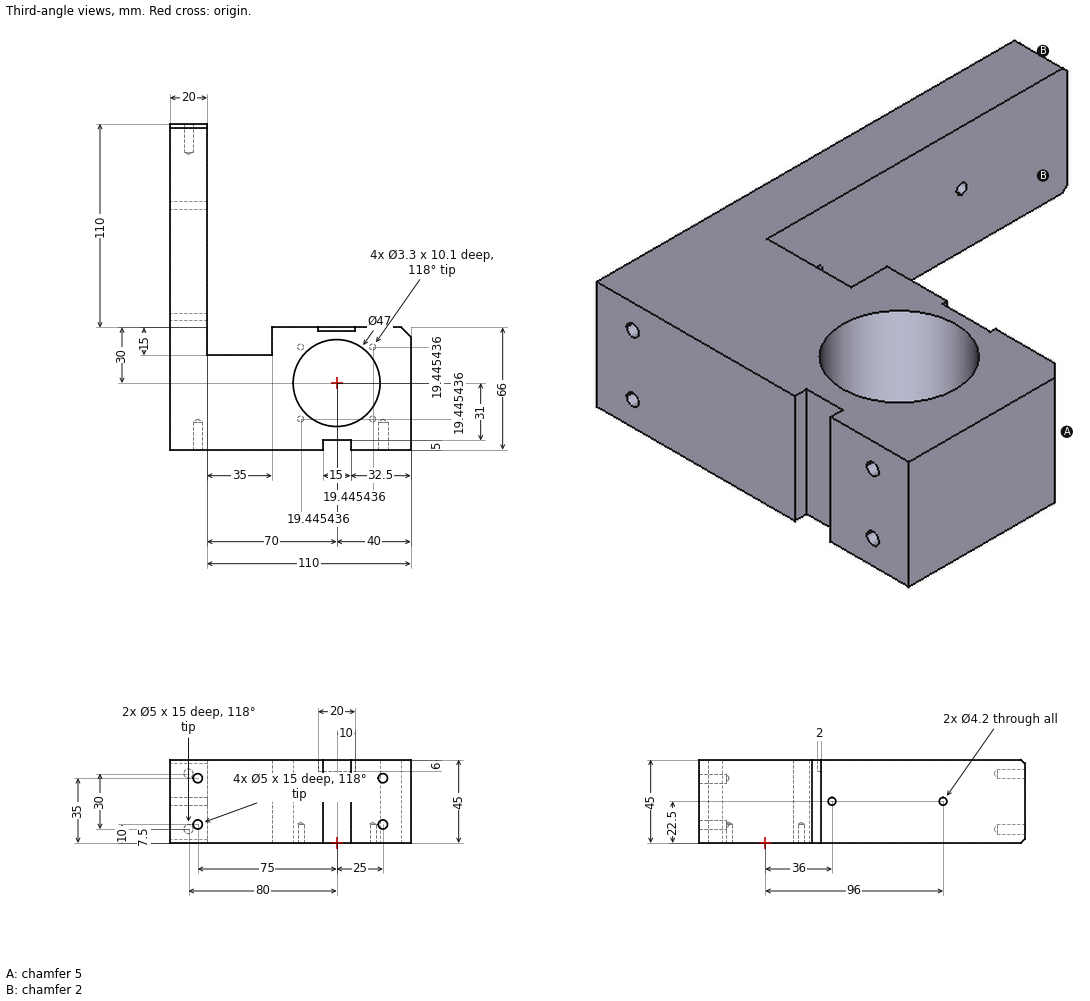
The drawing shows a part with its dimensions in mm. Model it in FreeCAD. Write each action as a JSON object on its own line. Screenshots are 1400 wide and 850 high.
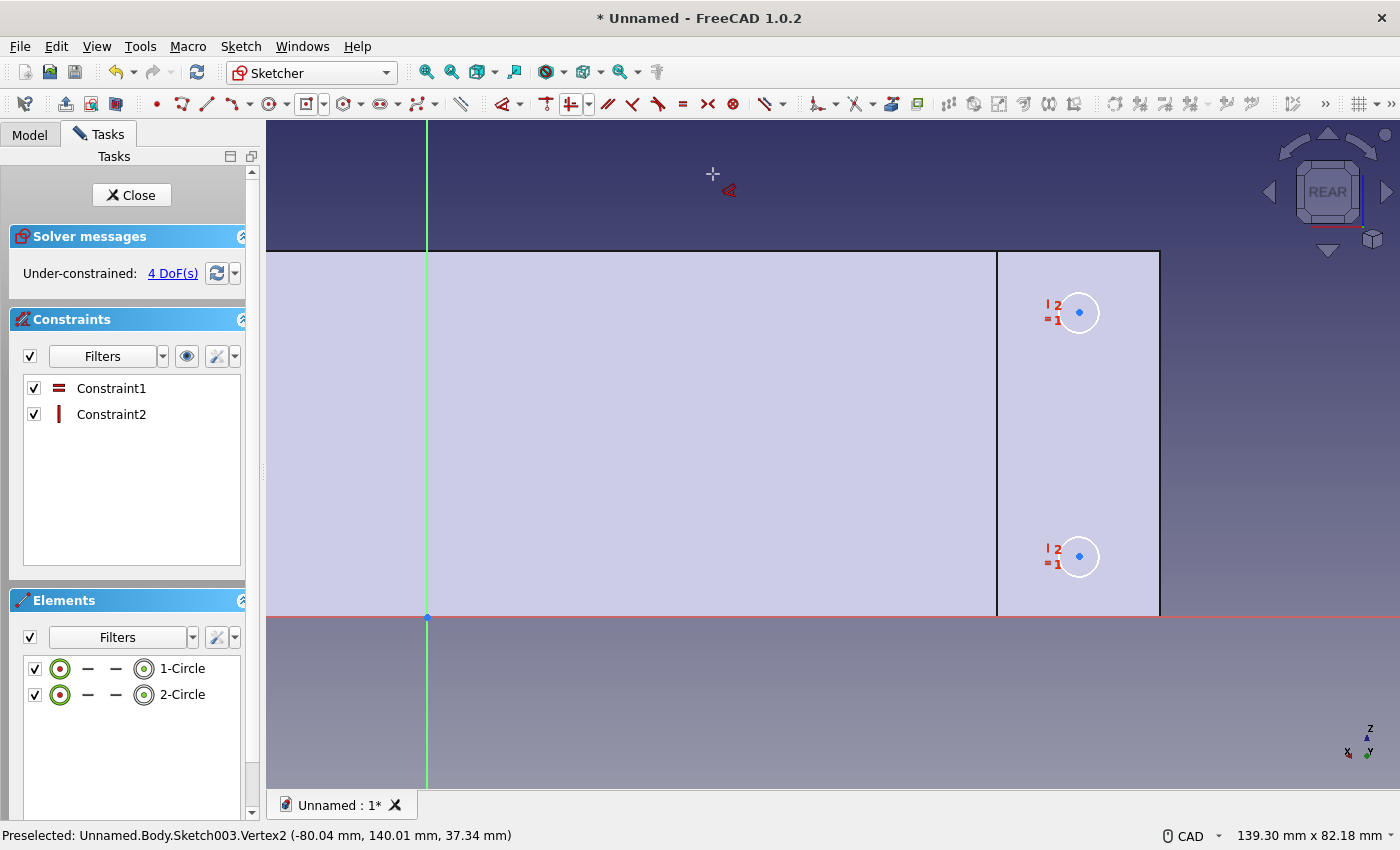
{"action": "left_click", "coordinate": [1093, 543]}
{"action": "left_click", "coordinate": [1116, 520]}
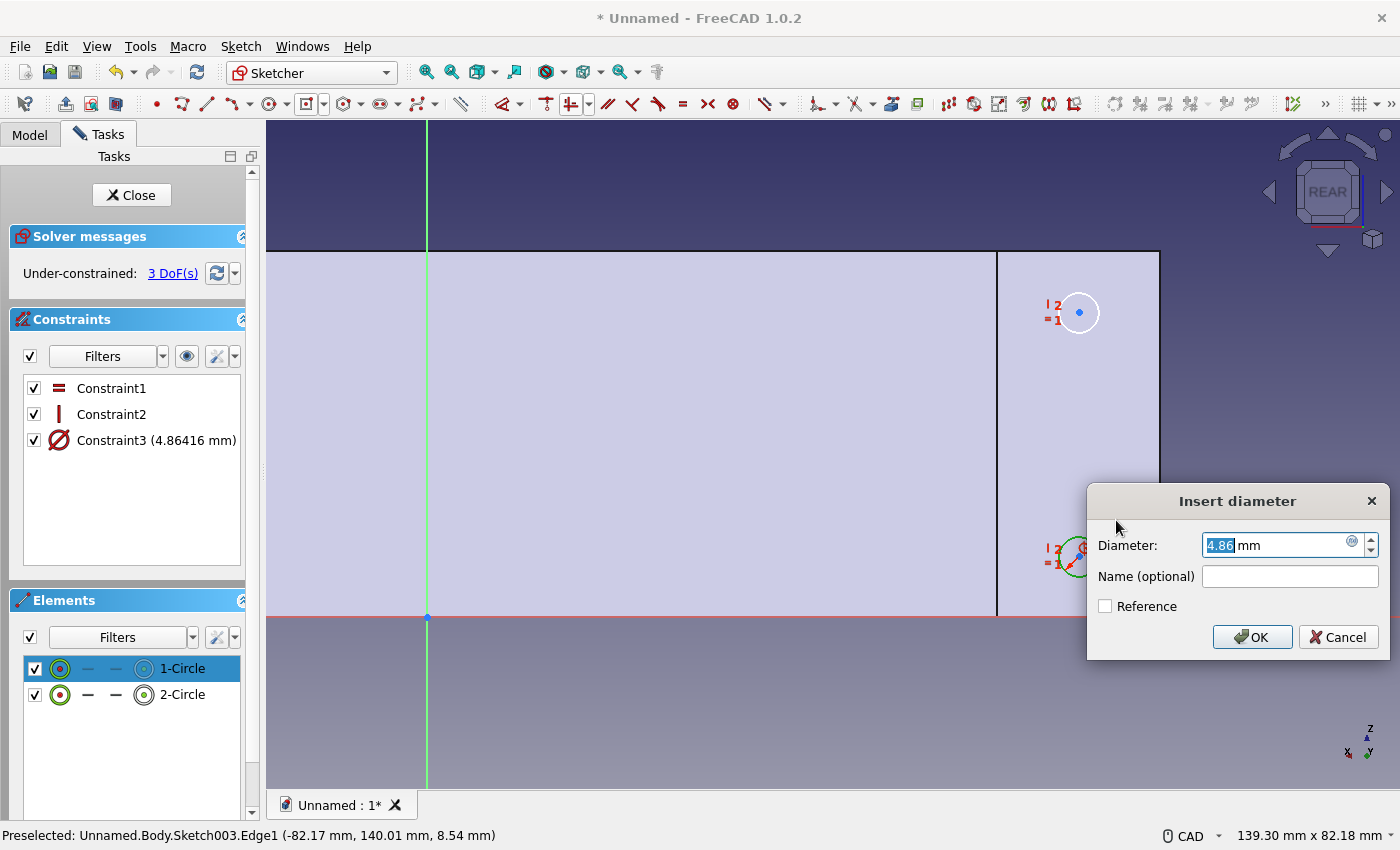
{"action": "type", "text": "5"}
{"action": "key", "text": "Return"}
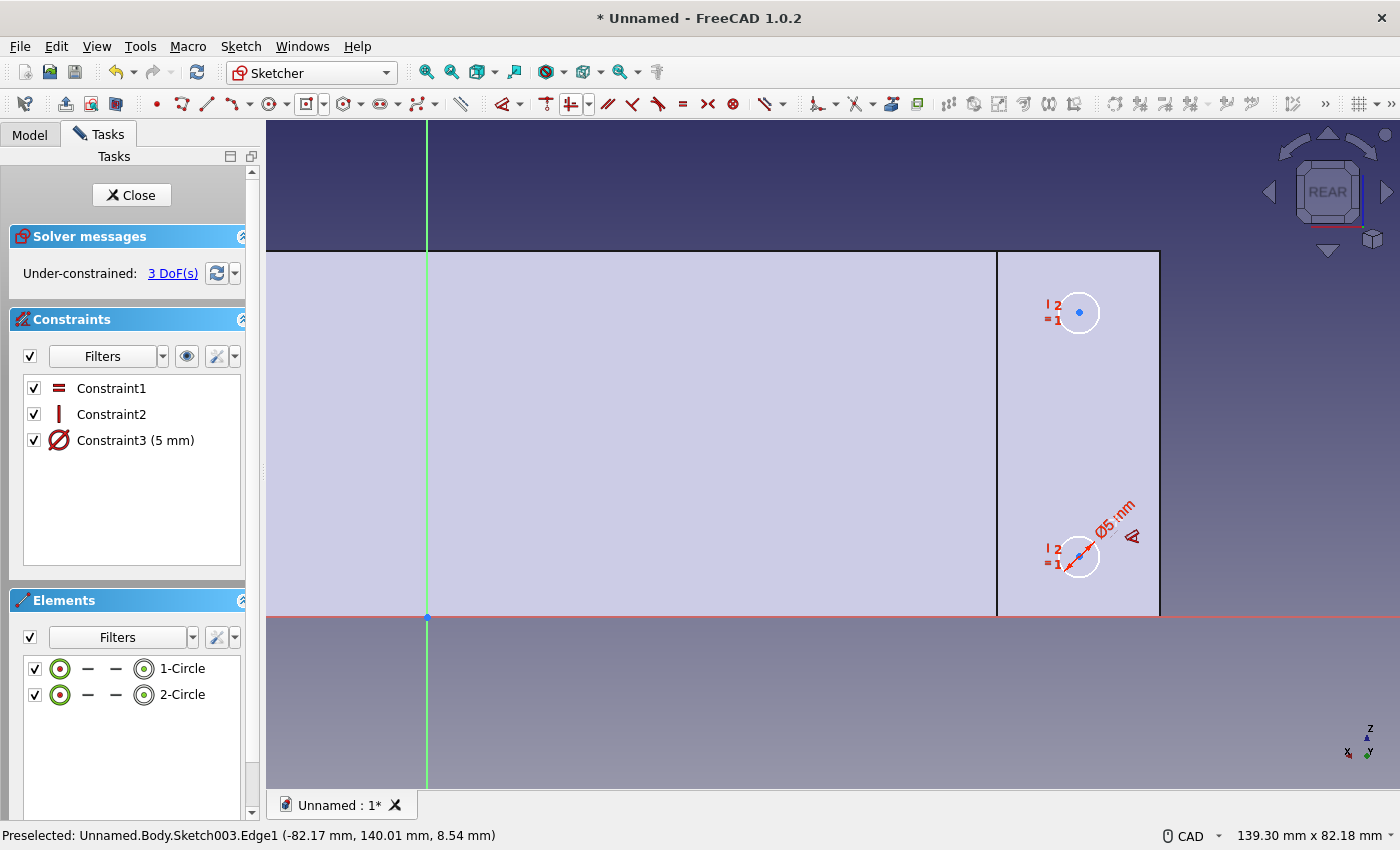
{"action": "left_click", "coordinate": [1079, 557]}
{"action": "left_click", "coordinate": [753, 651]}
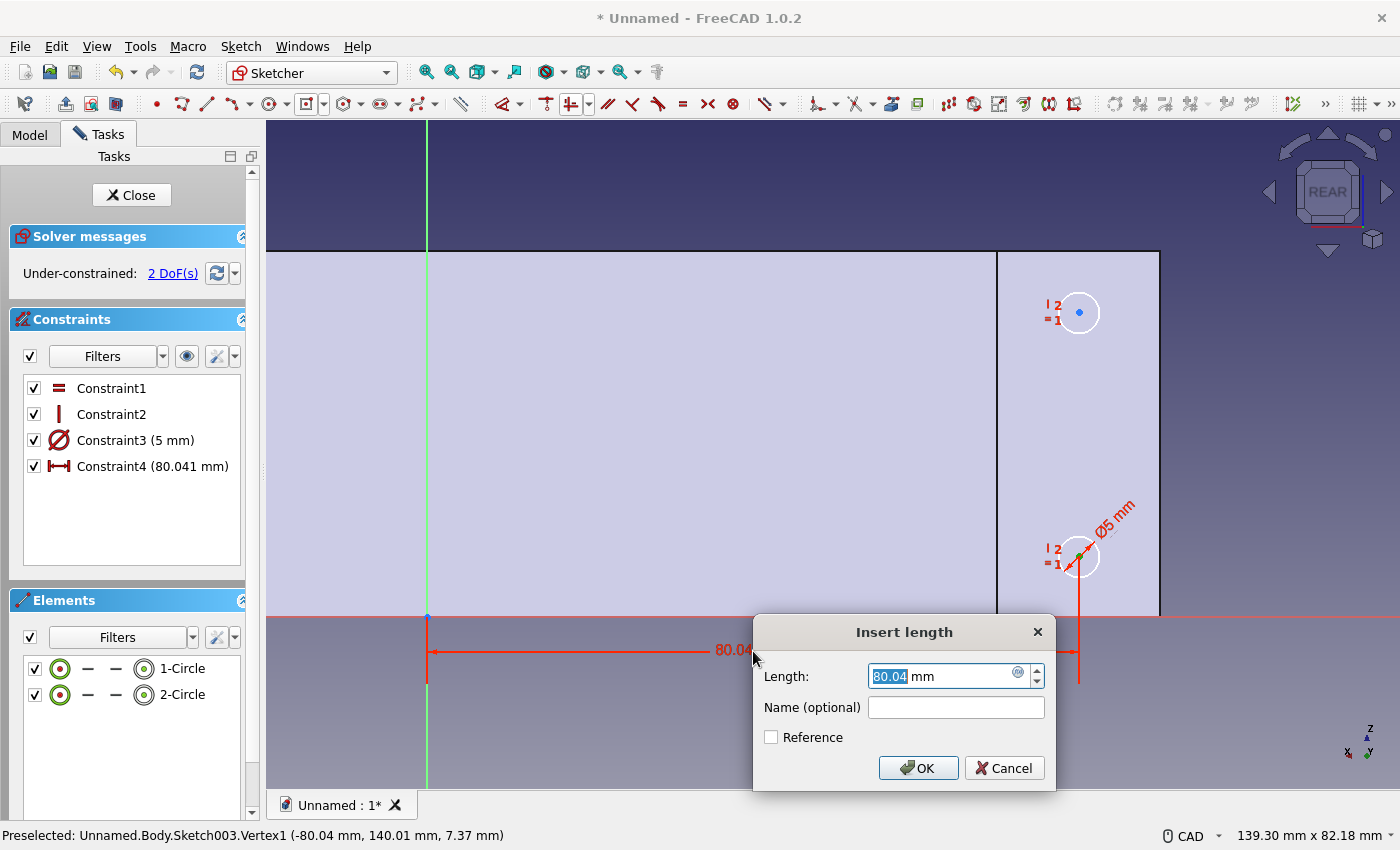
{"action": "type", "text": "80"}
{"action": "key", "text": "Return"}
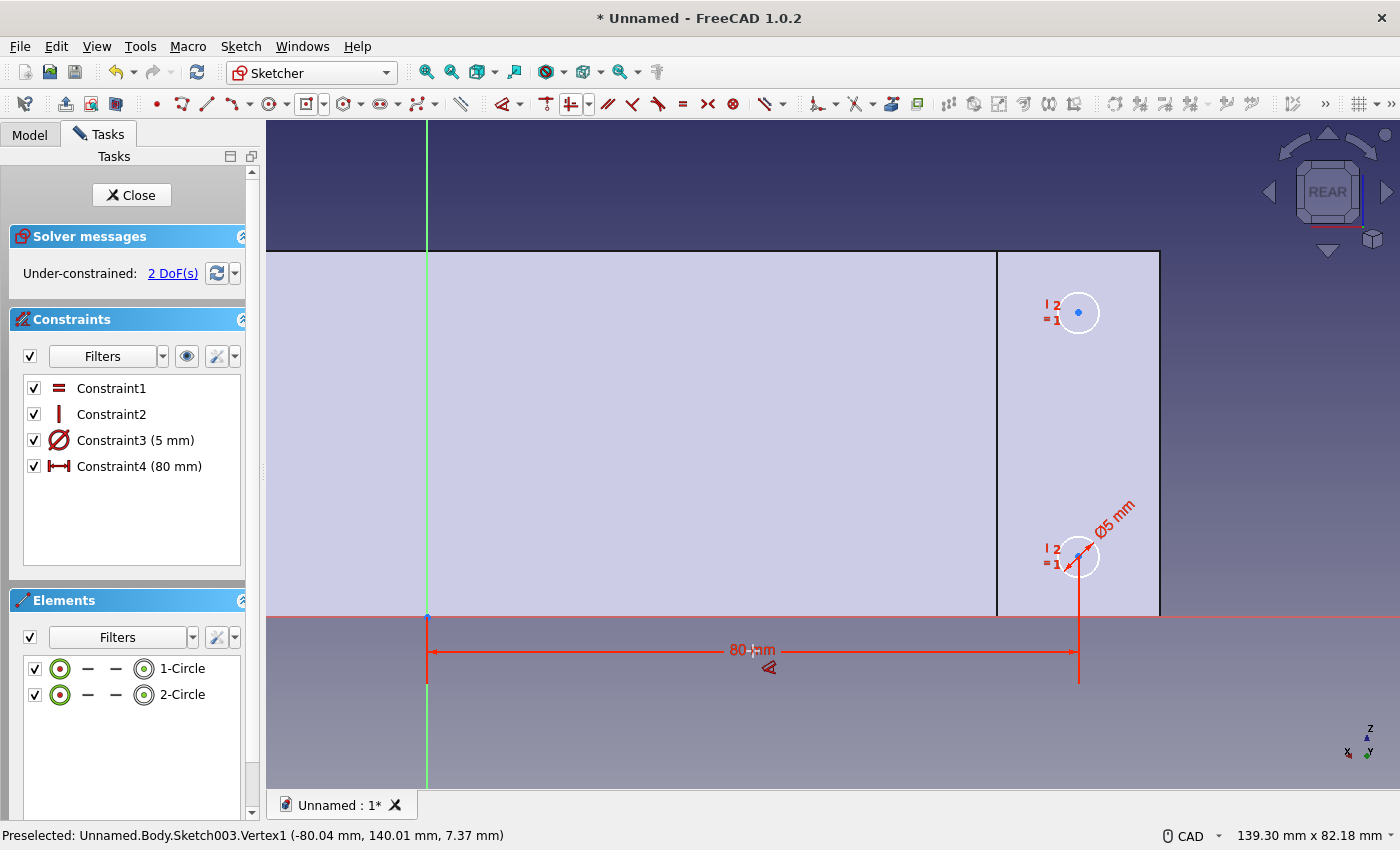
{"action": "left_click", "coordinate": [1079, 557]}
{"action": "left_click", "coordinate": [393, 587]}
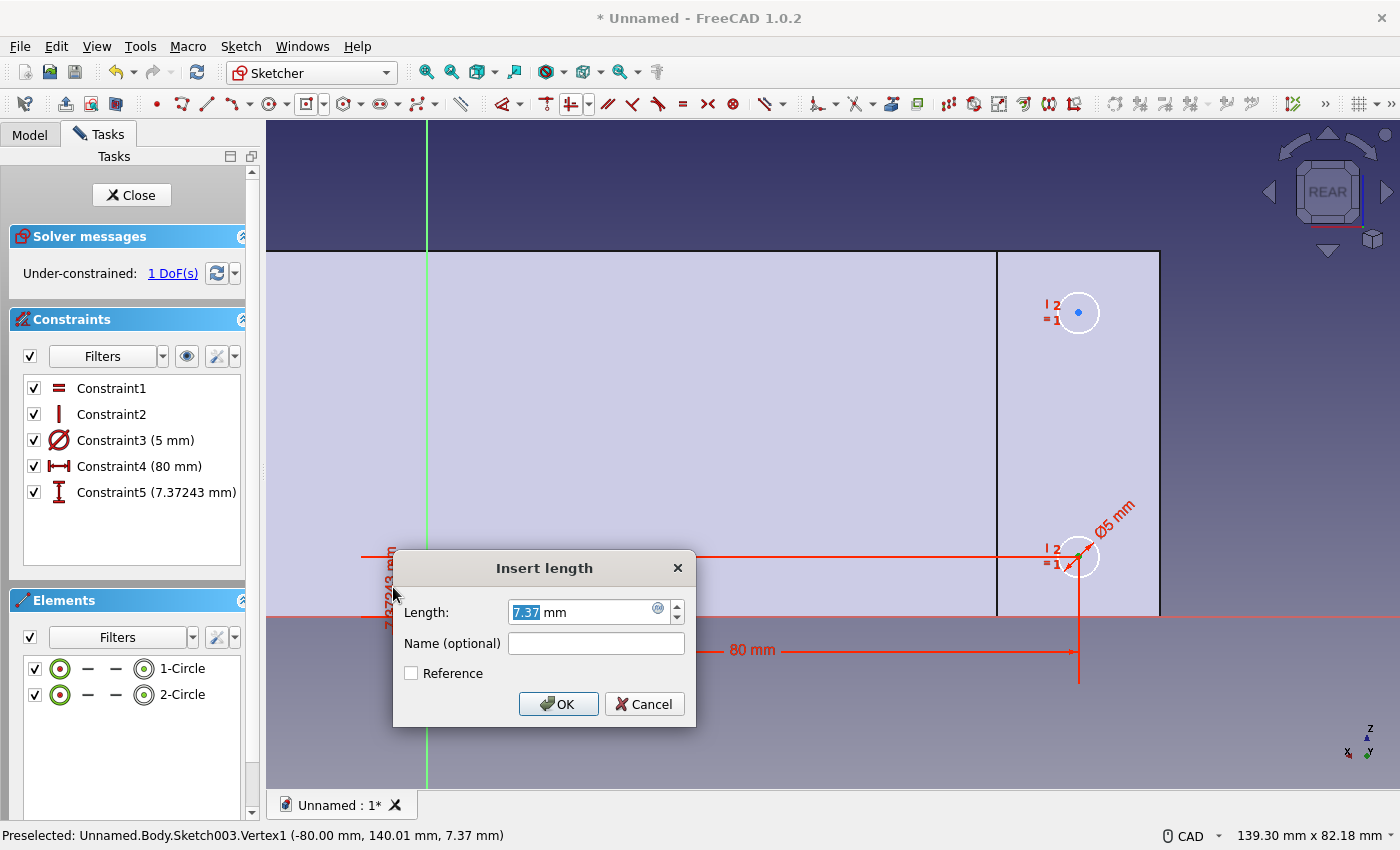
{"action": "type", "text": "7.5"}
{"action": "key", "text": "Return"}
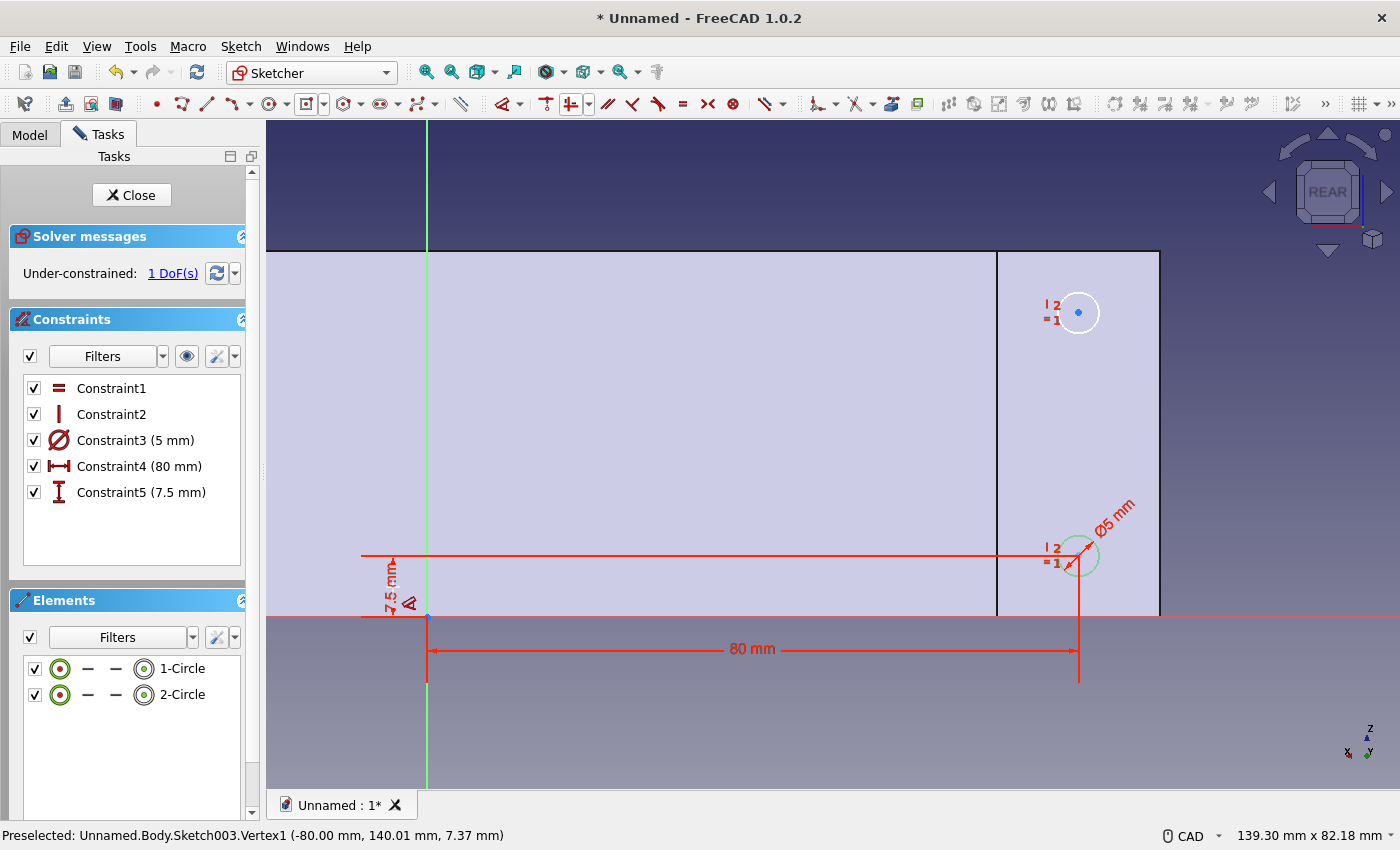
{"action": "left_click", "coordinate": [1079, 556]}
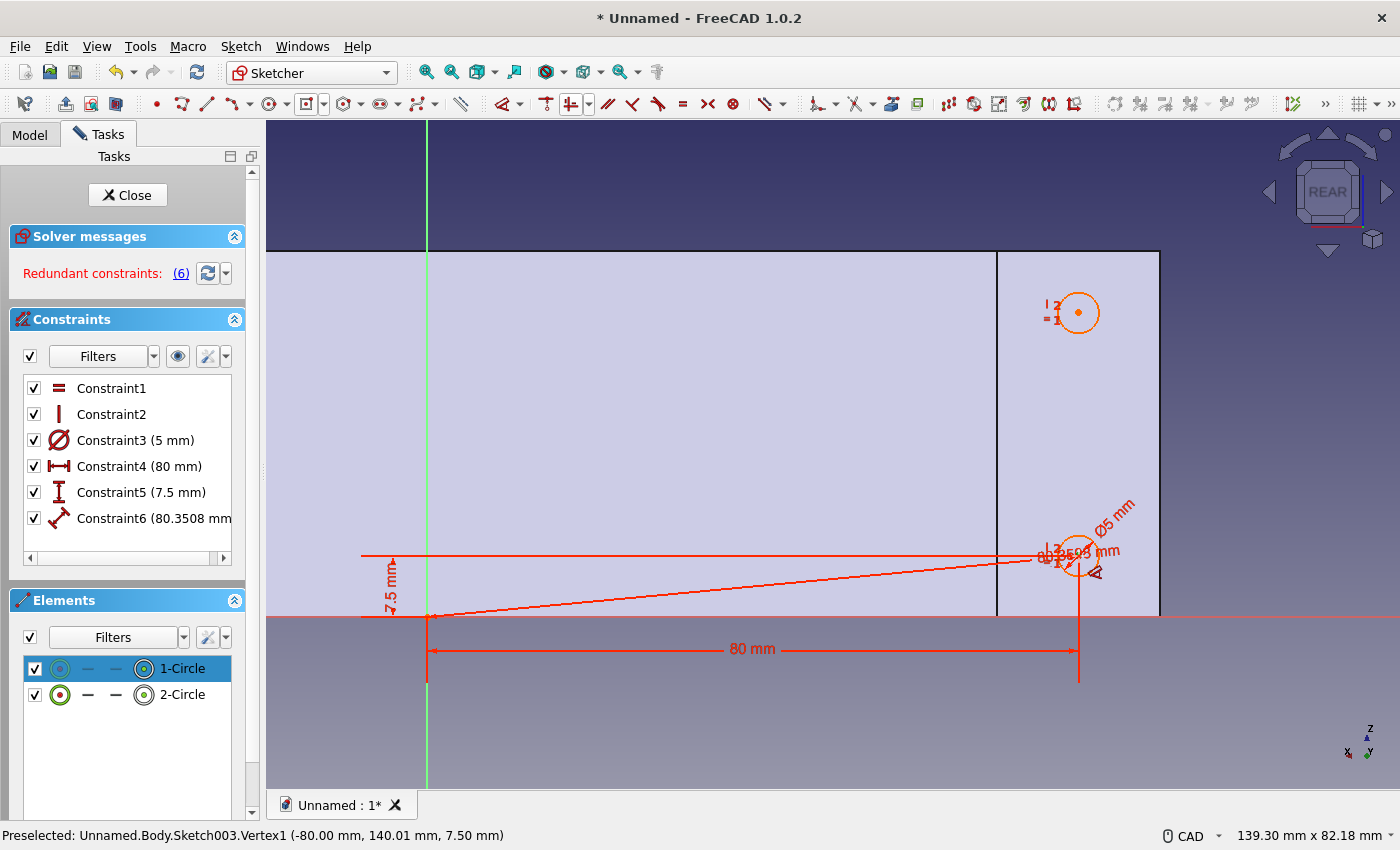
{"action": "left_click", "coordinate": [1079, 313]}
{"action": "left_click", "coordinate": [1113, 434]}